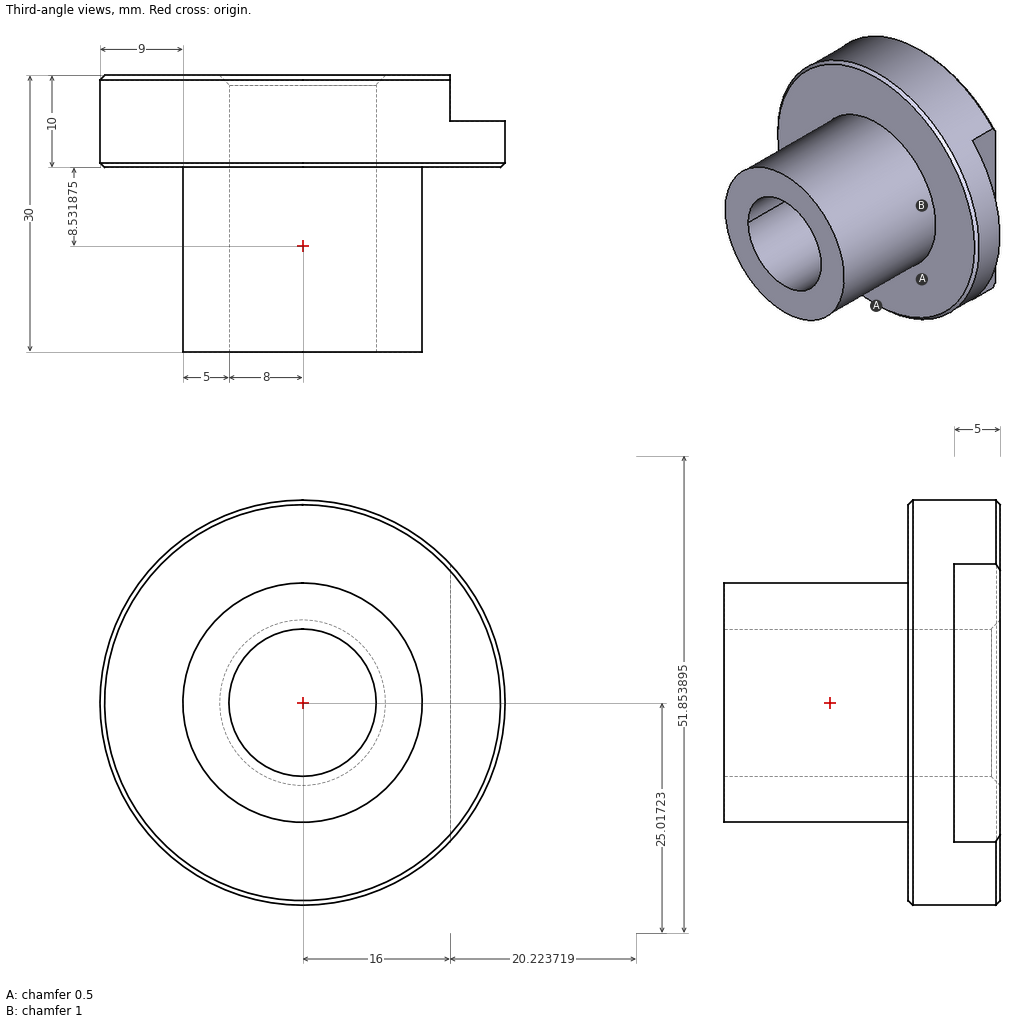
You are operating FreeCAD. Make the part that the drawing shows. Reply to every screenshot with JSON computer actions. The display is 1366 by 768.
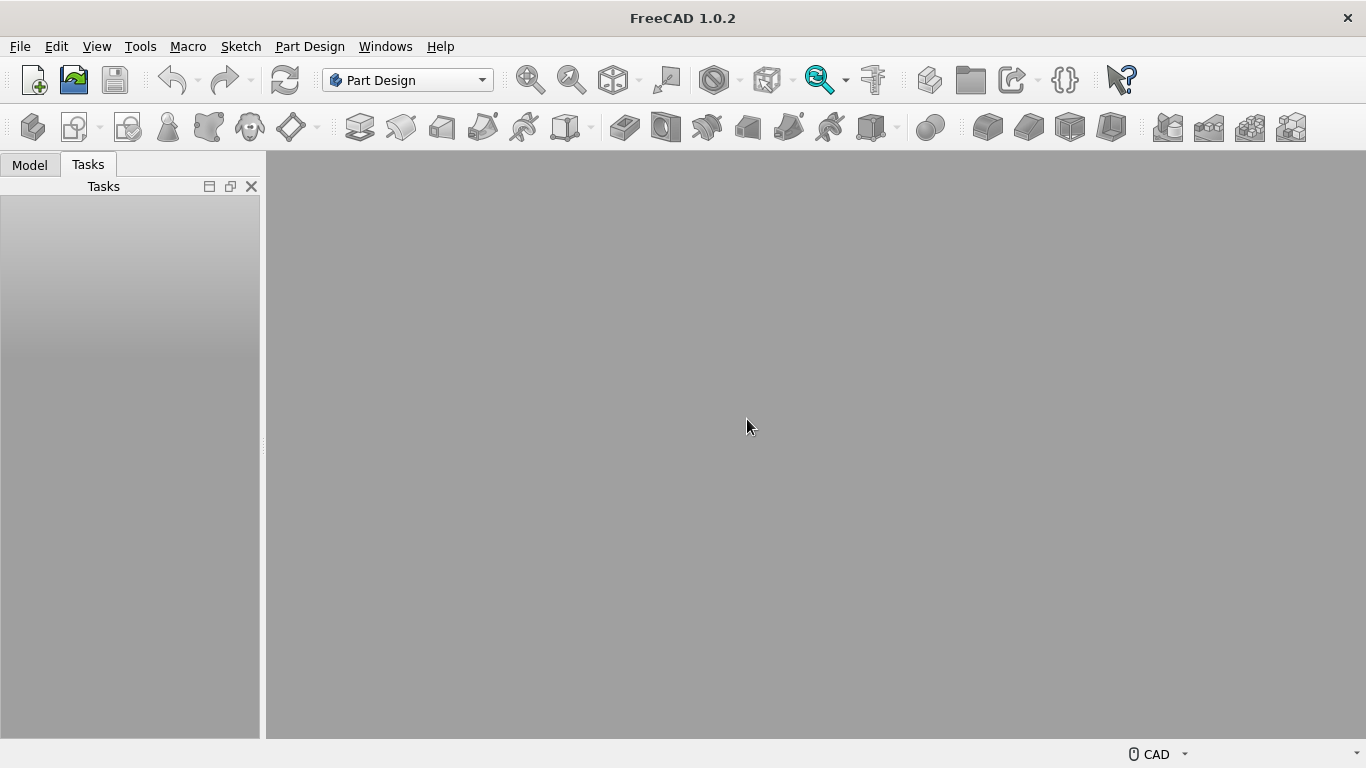
{"action": "left_click", "coordinate": [33, 80]}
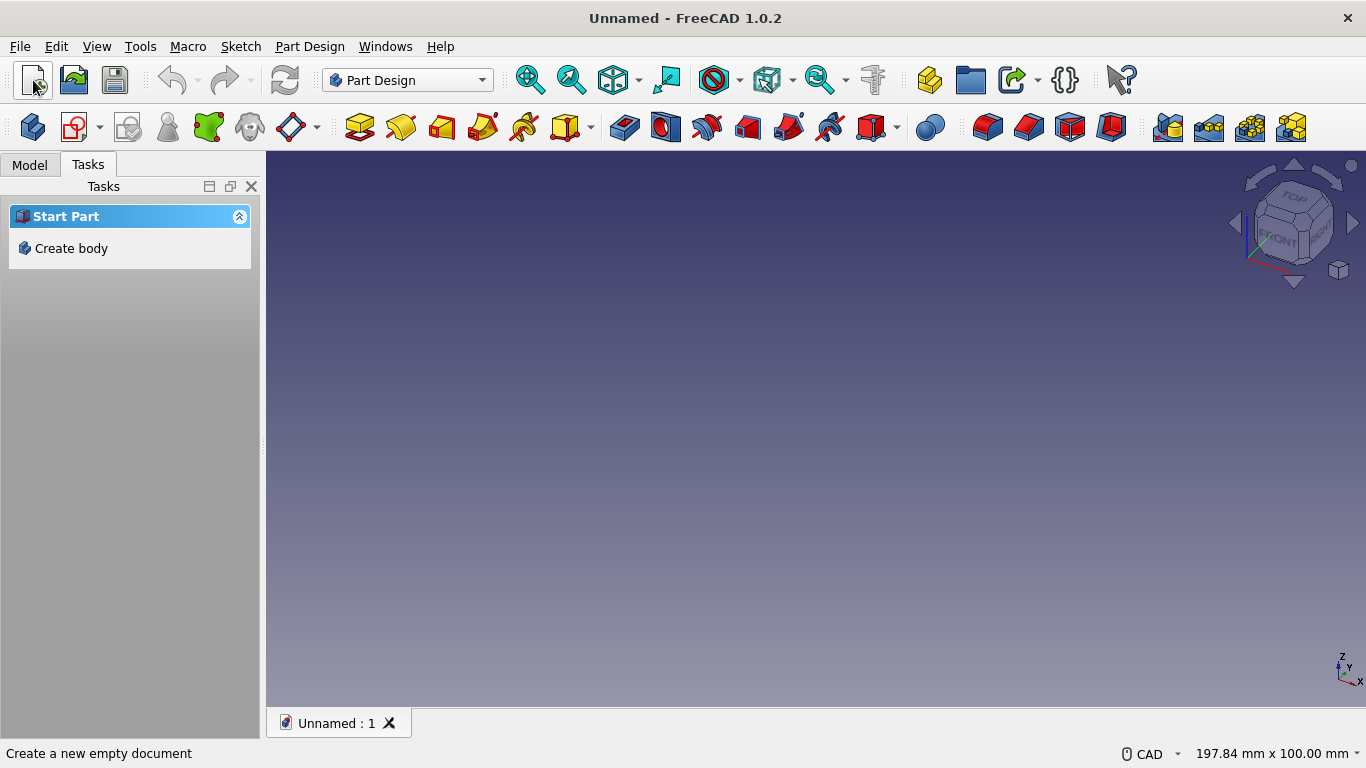
{"action": "left_click", "coordinate": [74, 128]}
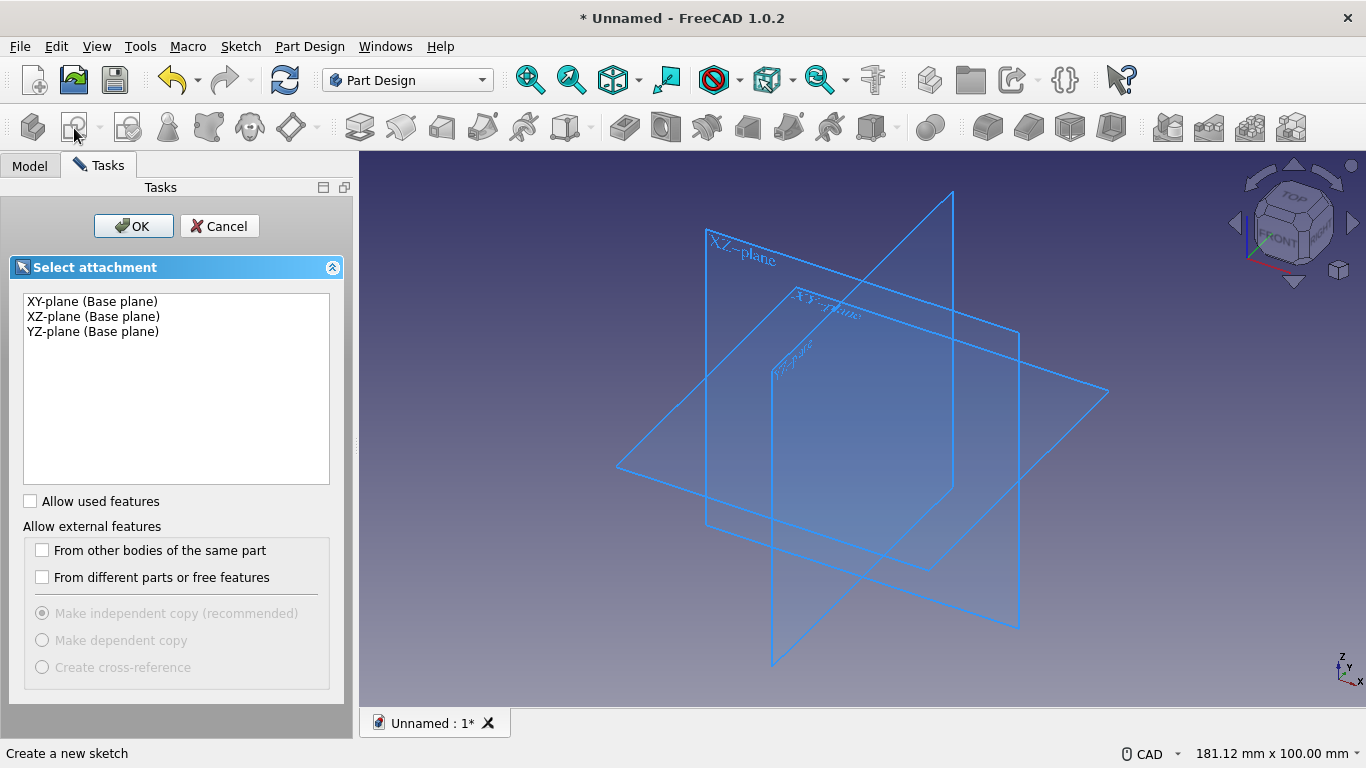
{"action": "left_click", "coordinate": [84, 302]}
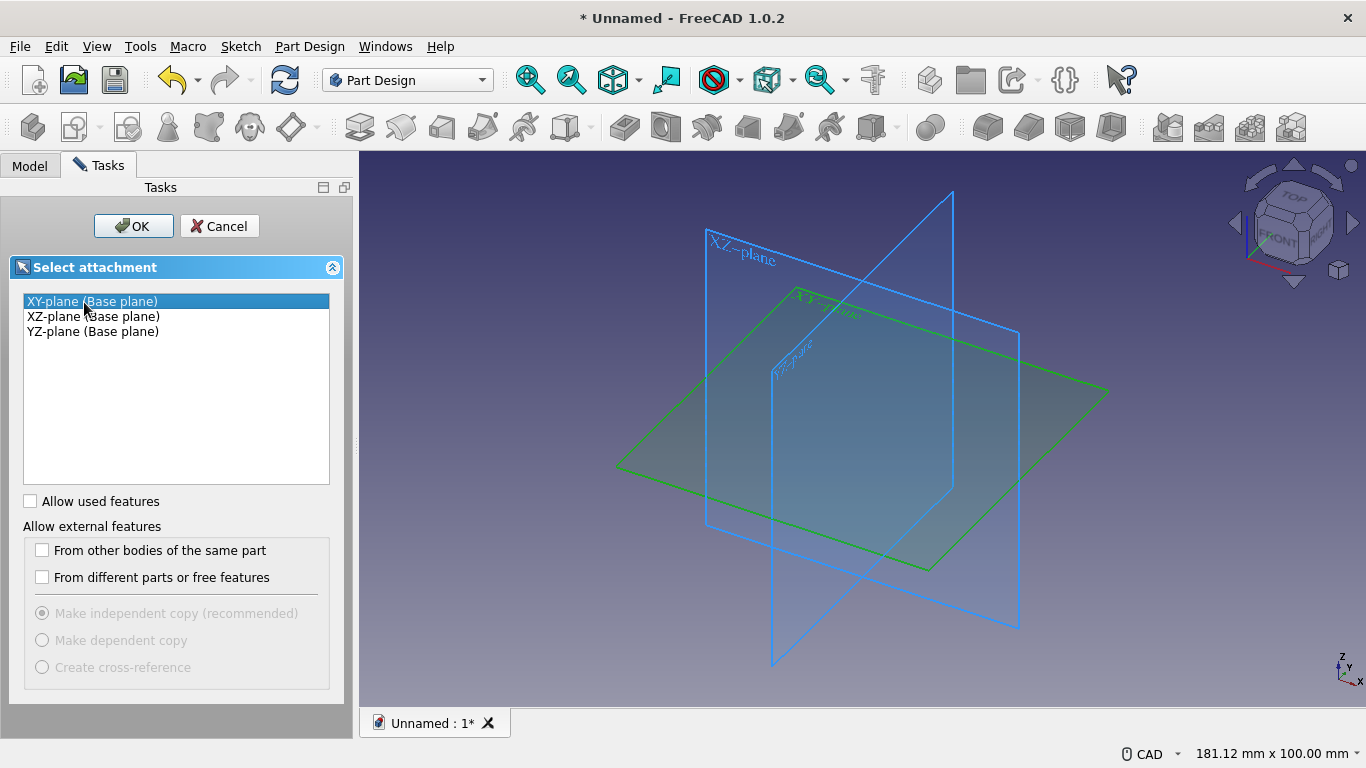
{"action": "left_click", "coordinate": [134, 226]}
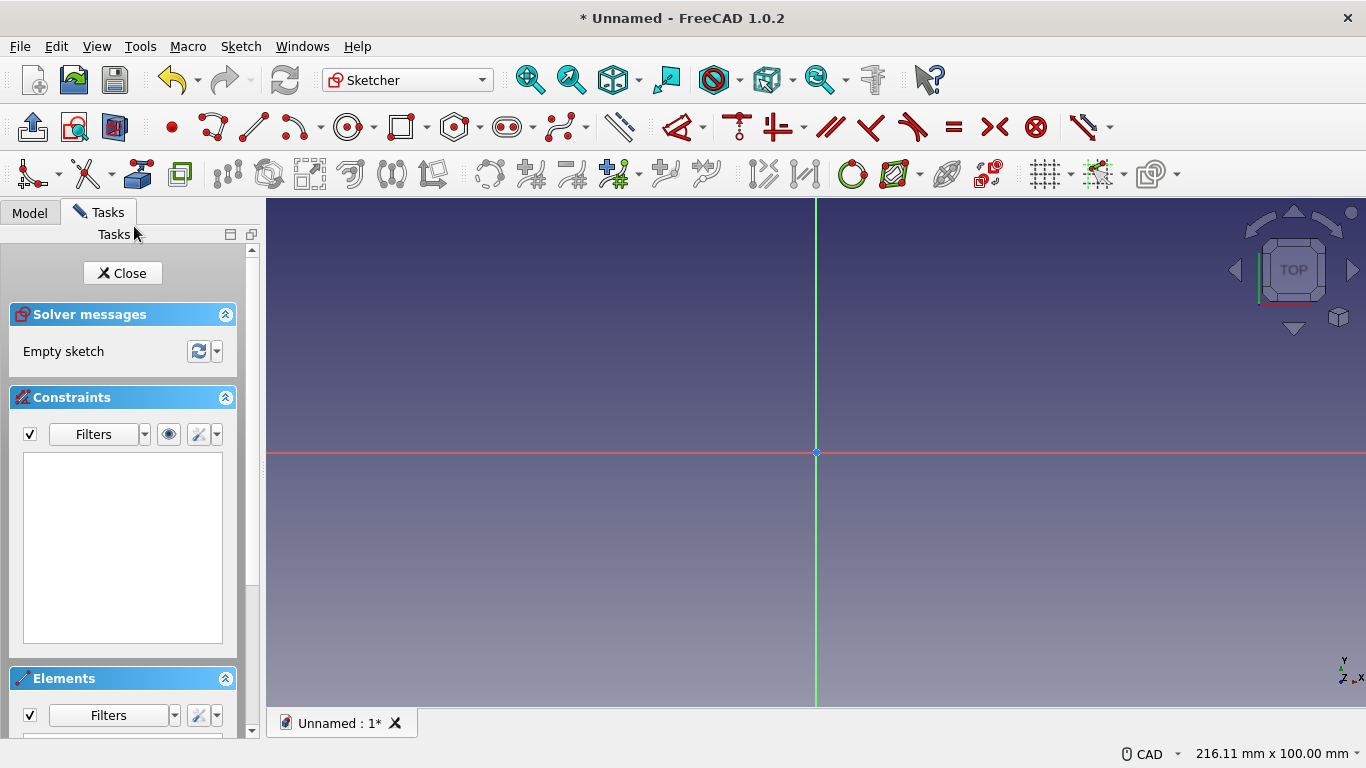
{"action": "scroll", "coordinate": [770, 420], "scroll_direction": "up", "scroll_amount": 4}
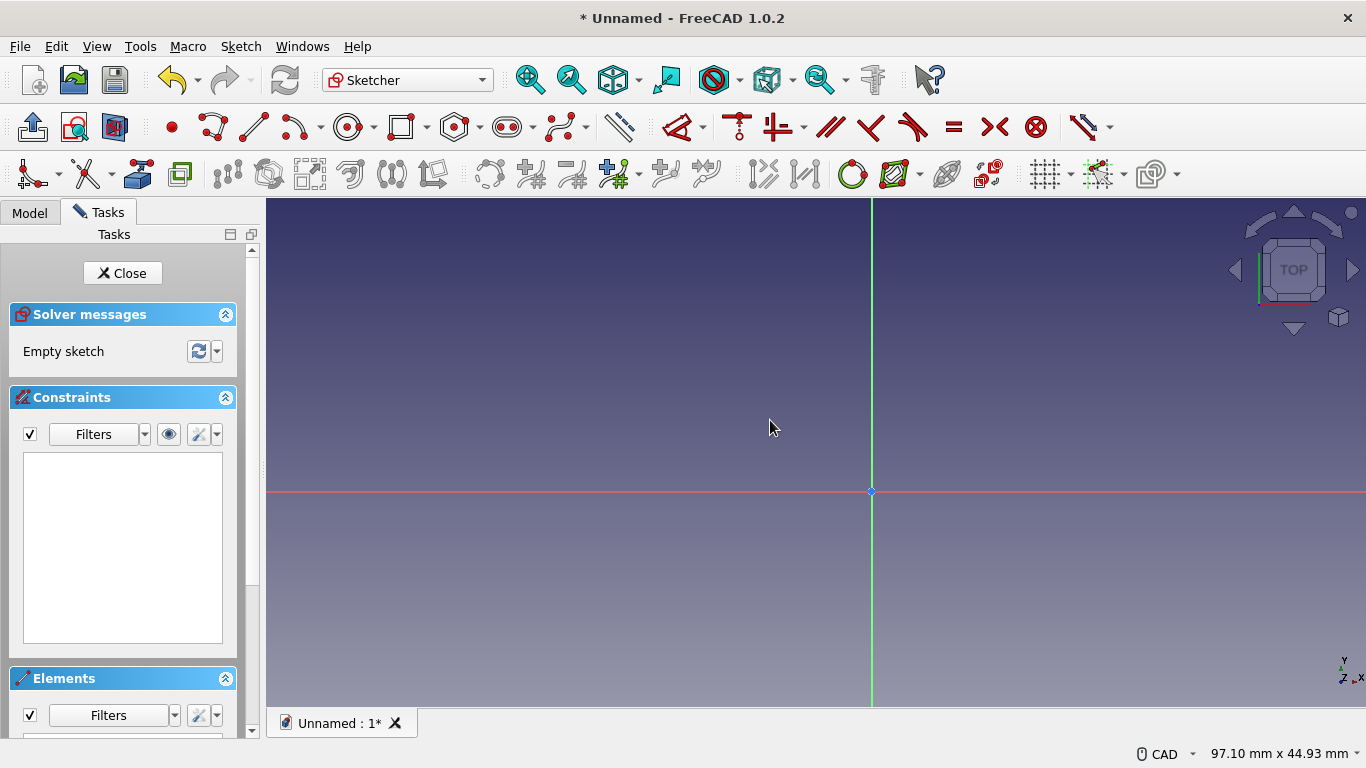
{"action": "left_click", "coordinate": [213, 128]}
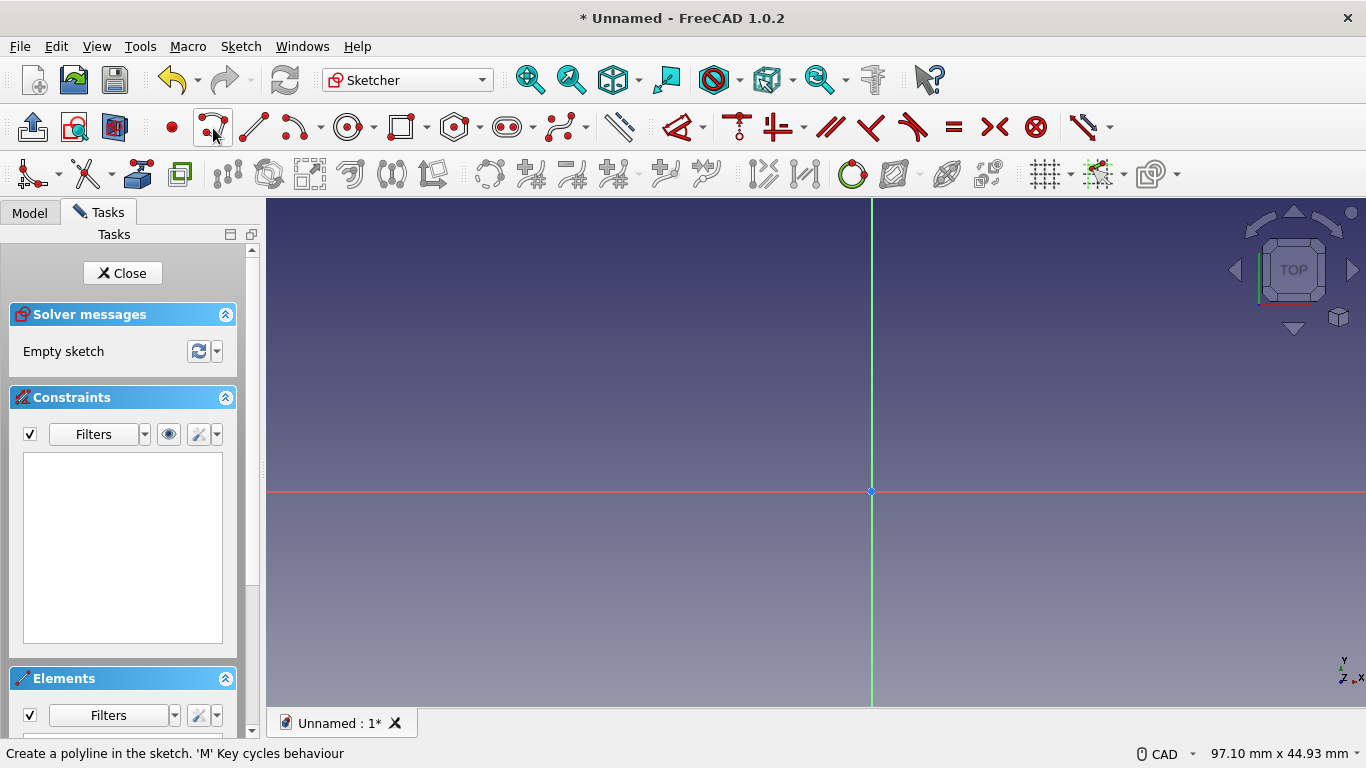
{"action": "left_click", "coordinate": [781, 622]}
{"action": "left_click", "coordinate": [781, 282]}
{"action": "left_click", "coordinate": [623, 282]}
{"action": "left_click", "coordinate": [623, 395]}
{"action": "left_click", "coordinate": [725, 395]}
{"action": "left_click", "coordinate": [725, 622]}
{"action": "left_click", "coordinate": [781, 623]}
{"action": "key", "text": "Escape"}
{"action": "key", "text": "Escape"}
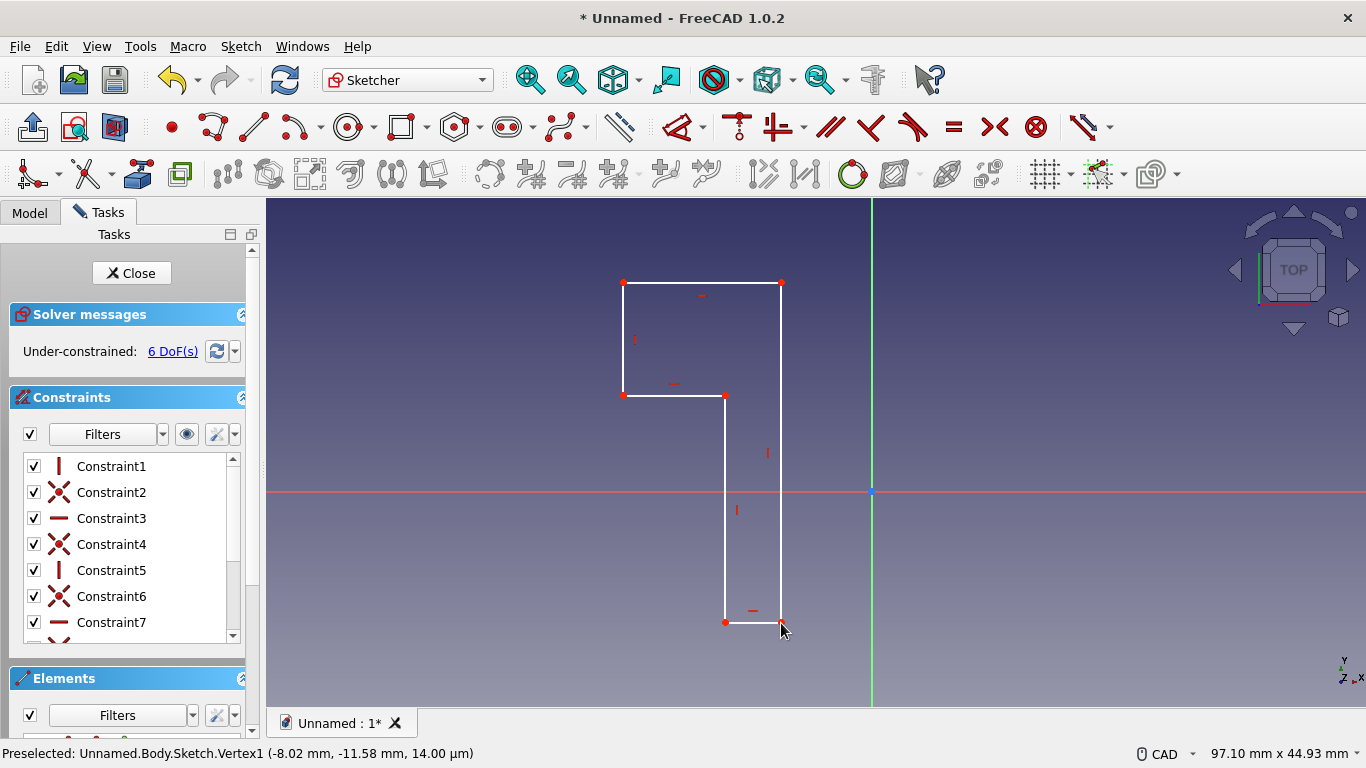
{"action": "left_click", "coordinate": [676, 128]}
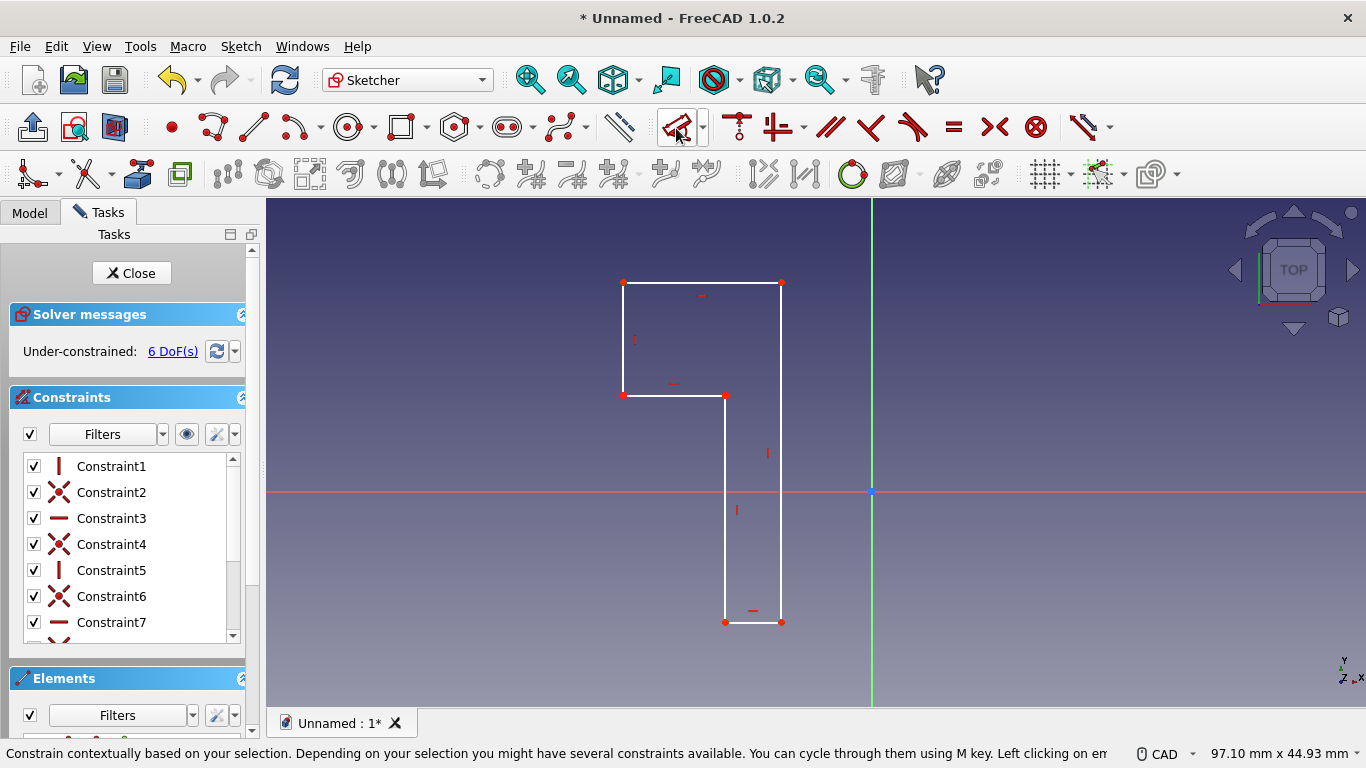
{"action": "left_click", "coordinate": [654, 396]}
{"action": "left_click", "coordinate": [674, 362]}